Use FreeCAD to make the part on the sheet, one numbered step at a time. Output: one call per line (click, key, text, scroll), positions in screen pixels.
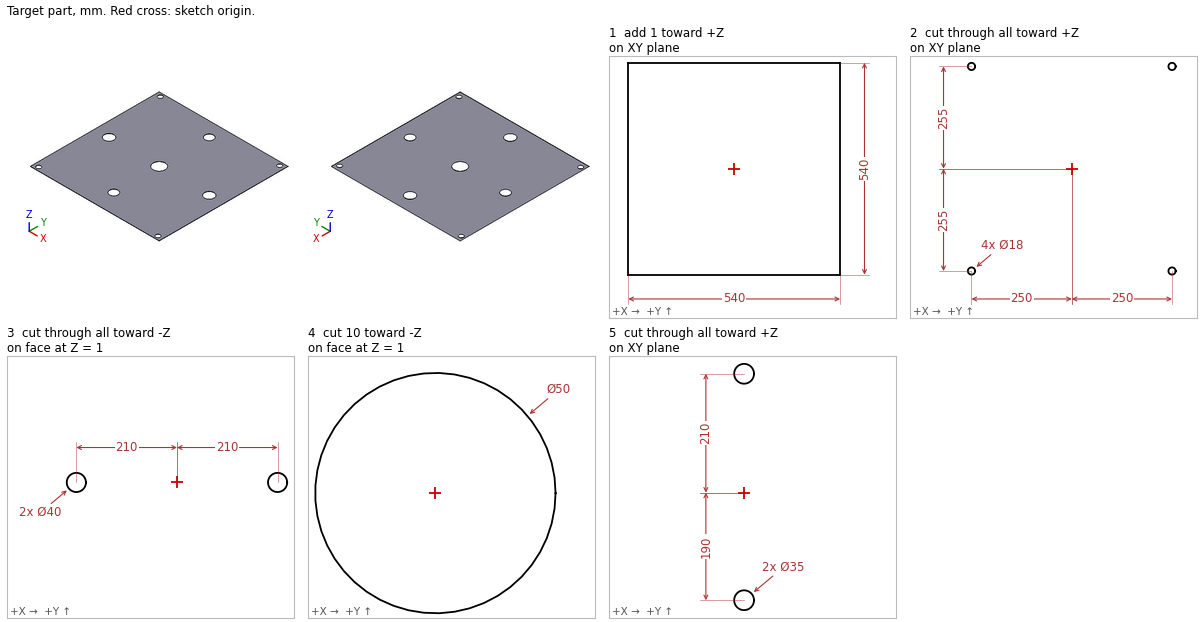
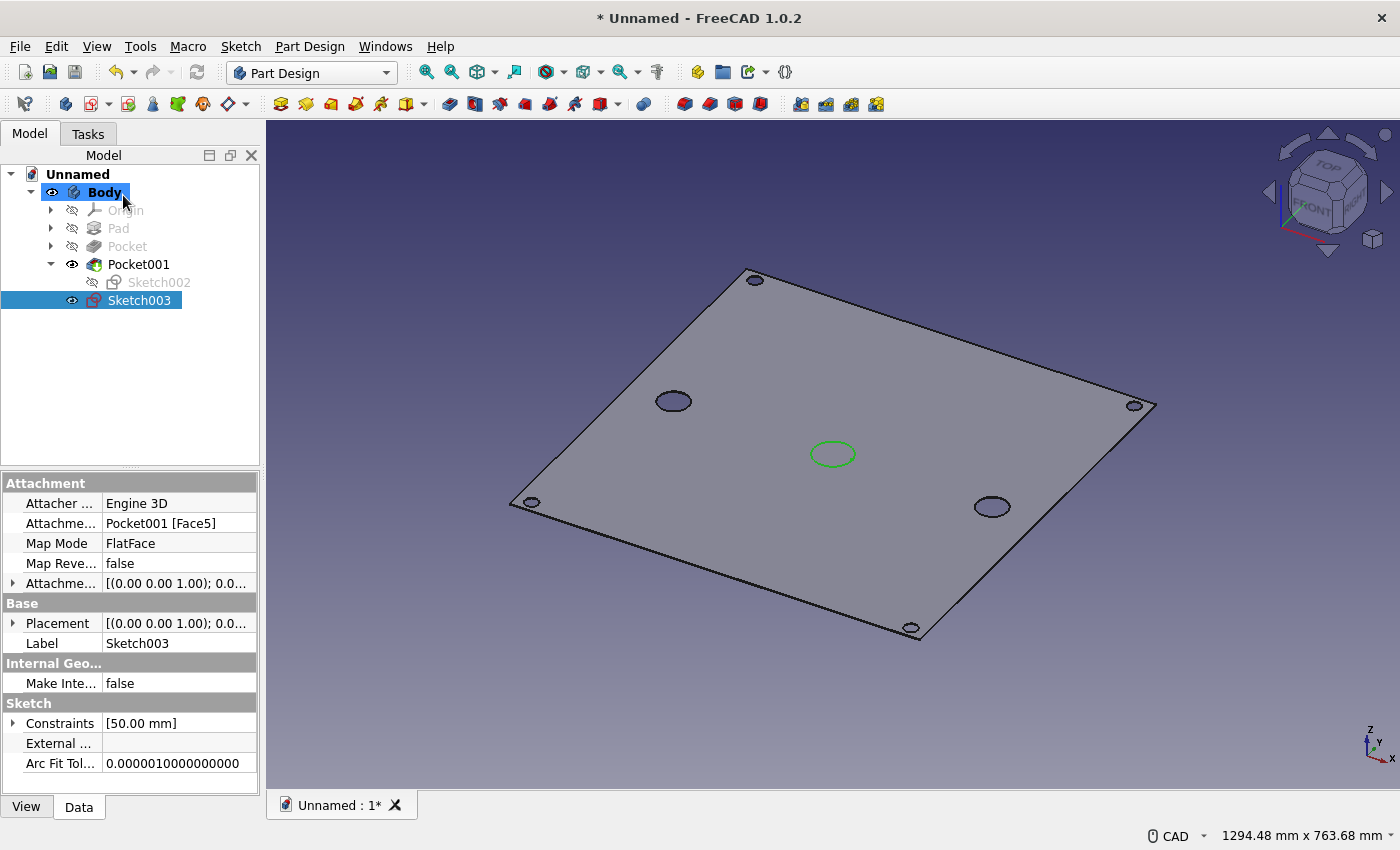
click(450, 104)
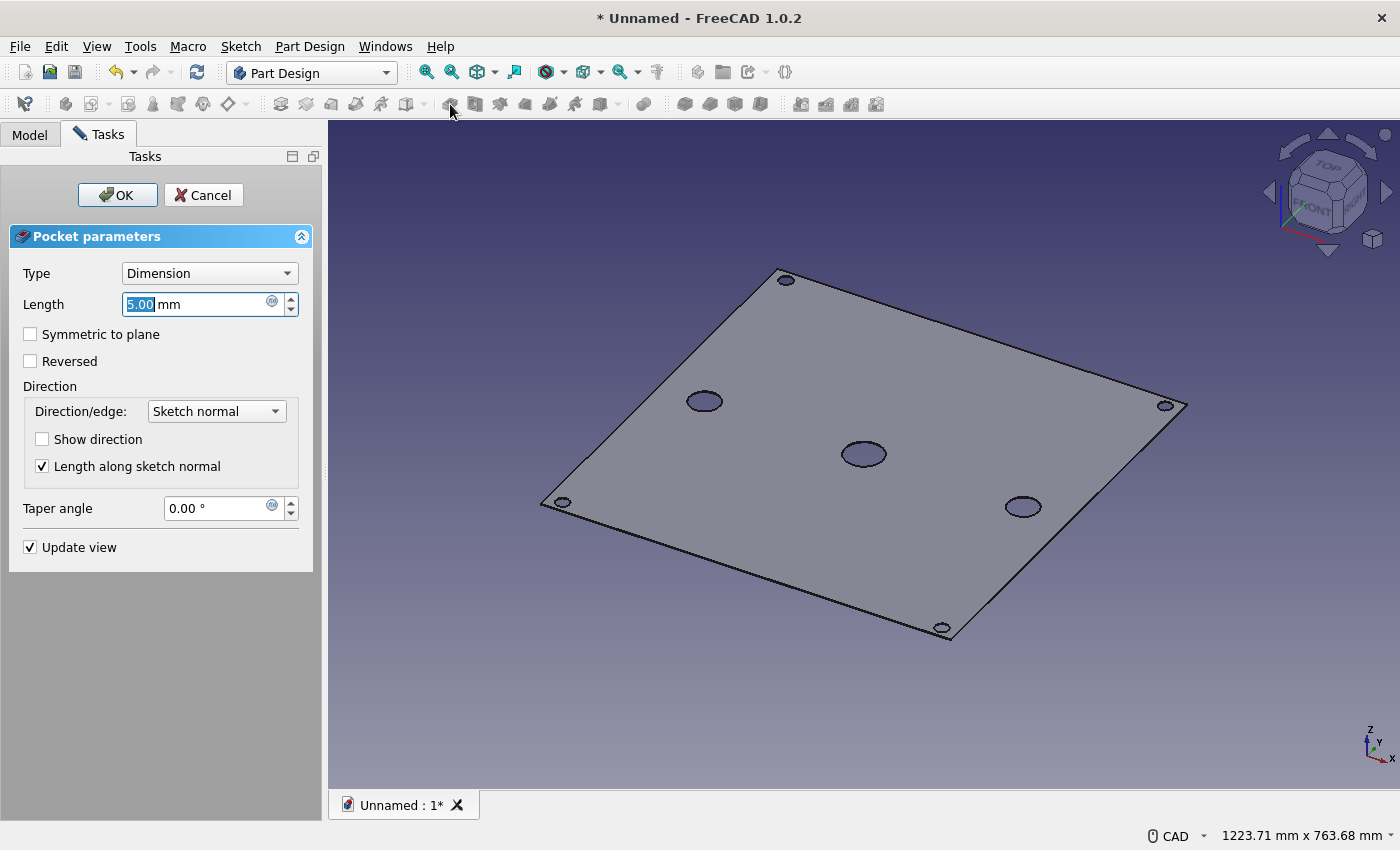
text(10)
key(Tab)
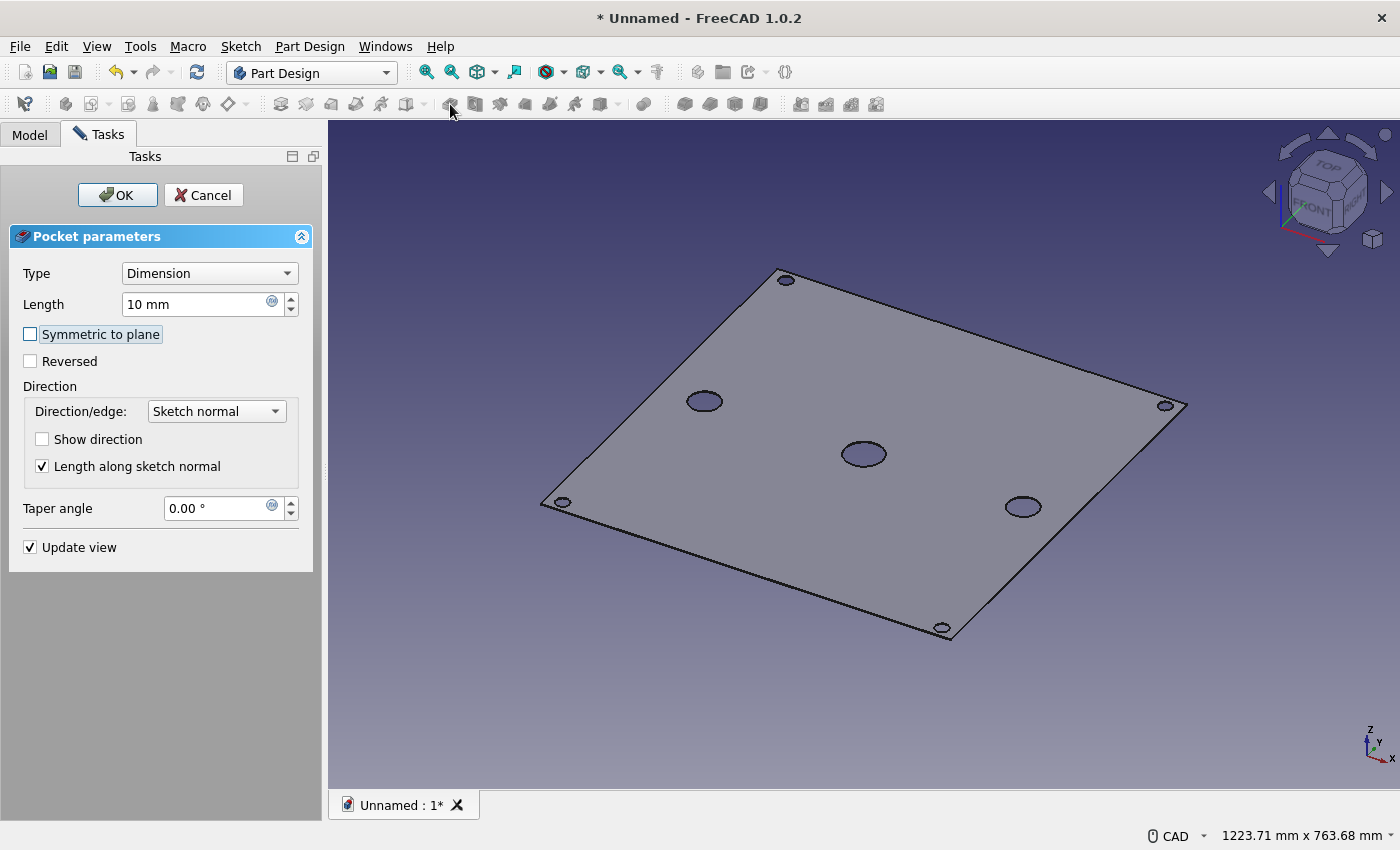
click(118, 195)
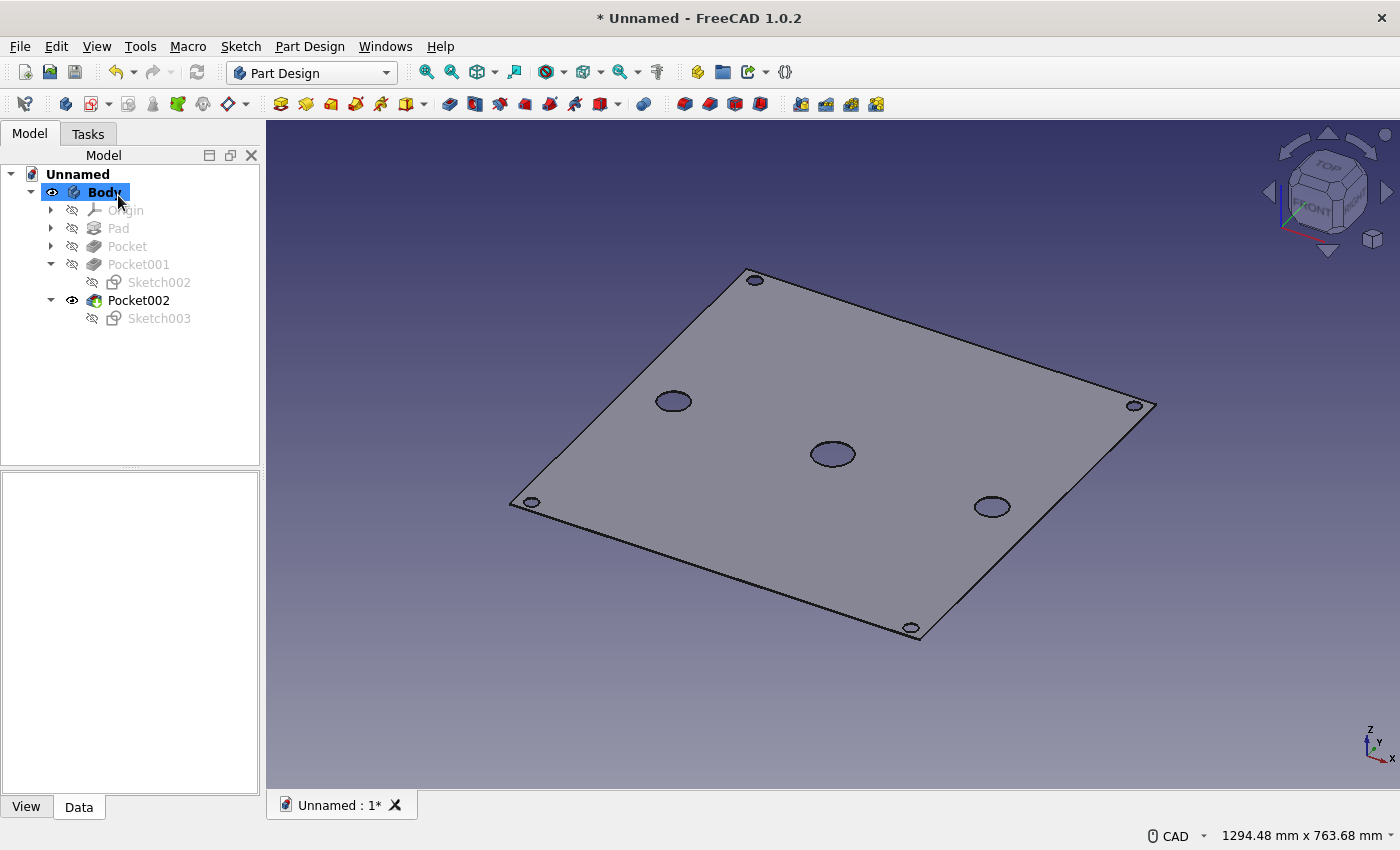
click(90, 104)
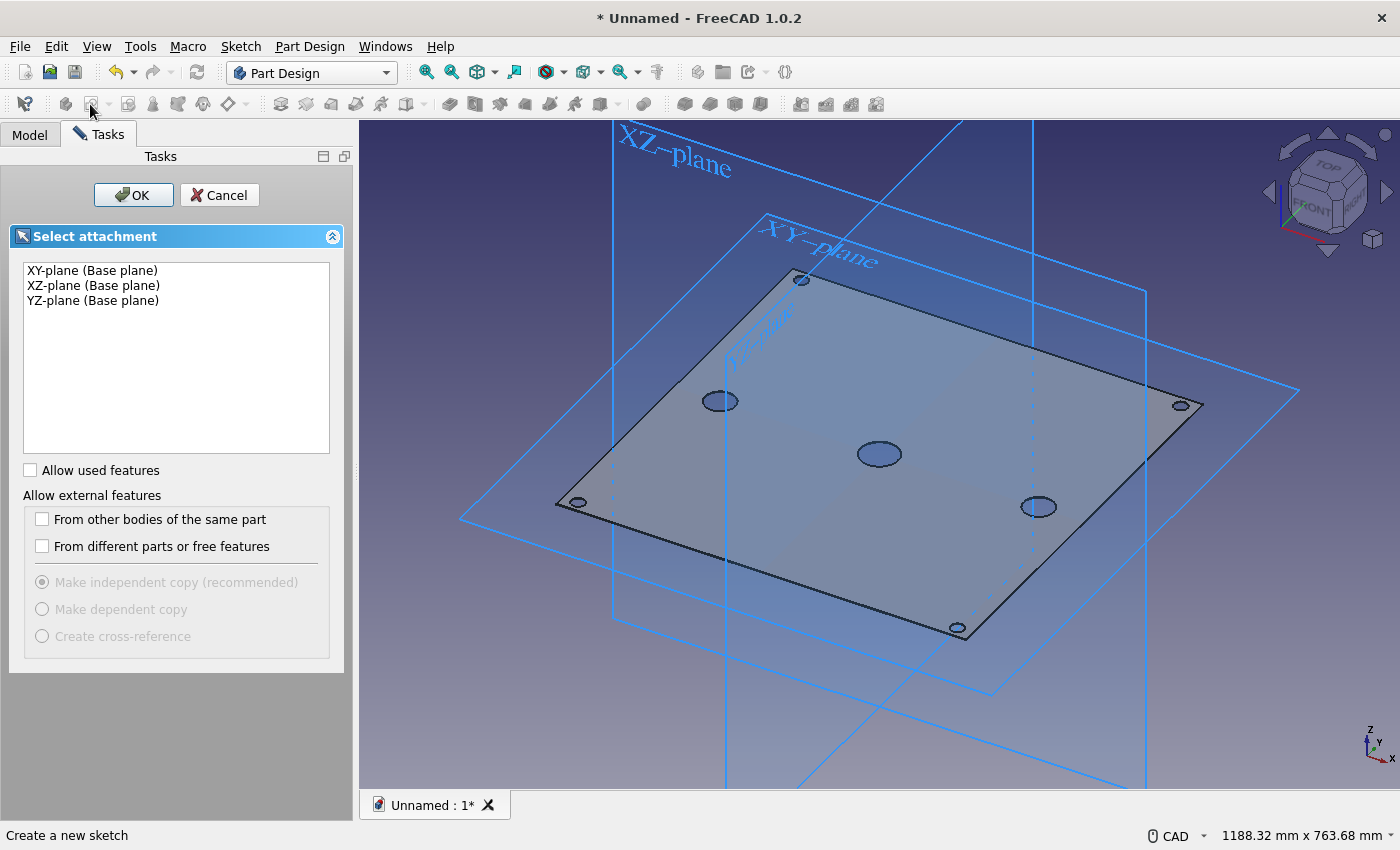
click(84, 270)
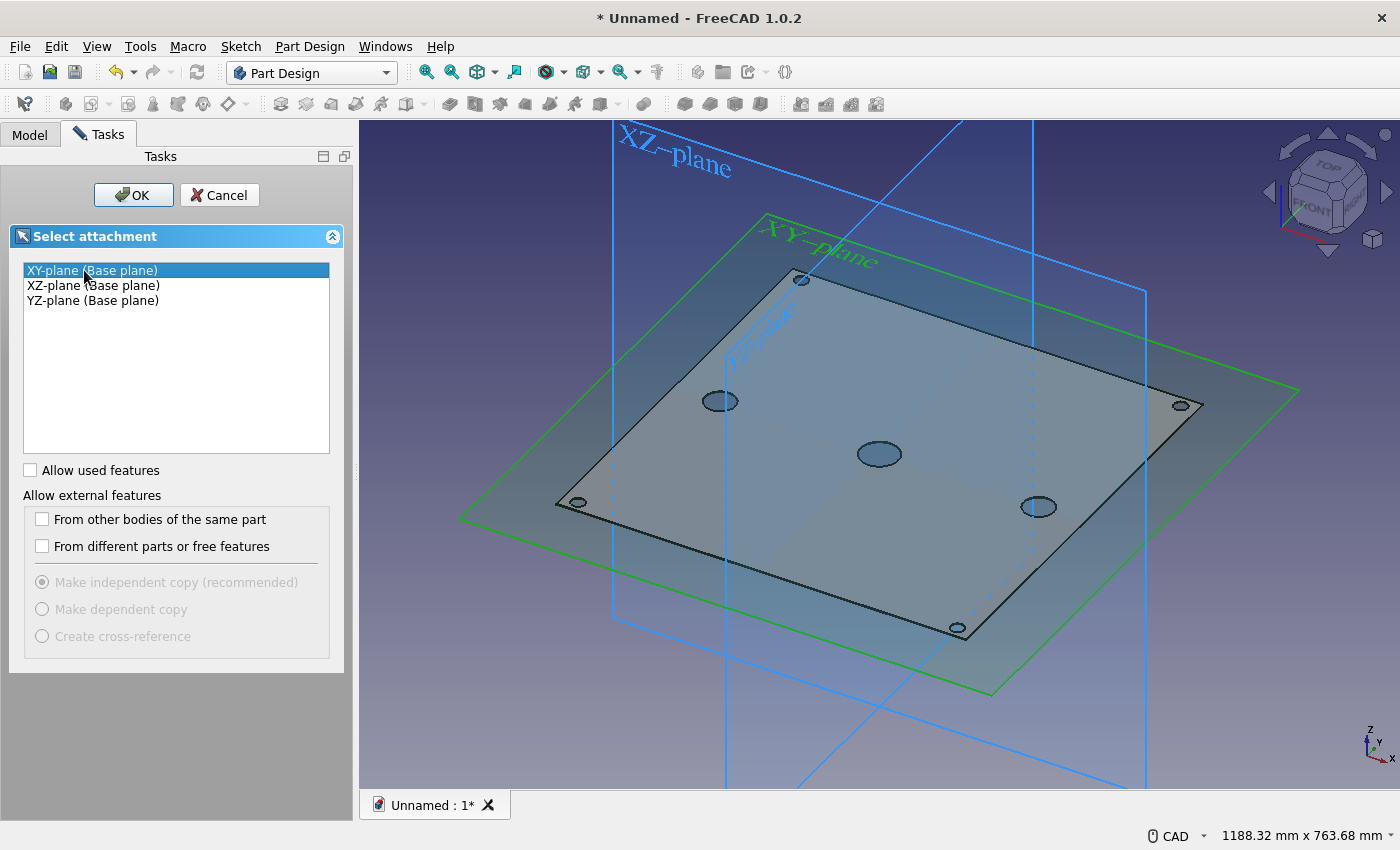
click(134, 195)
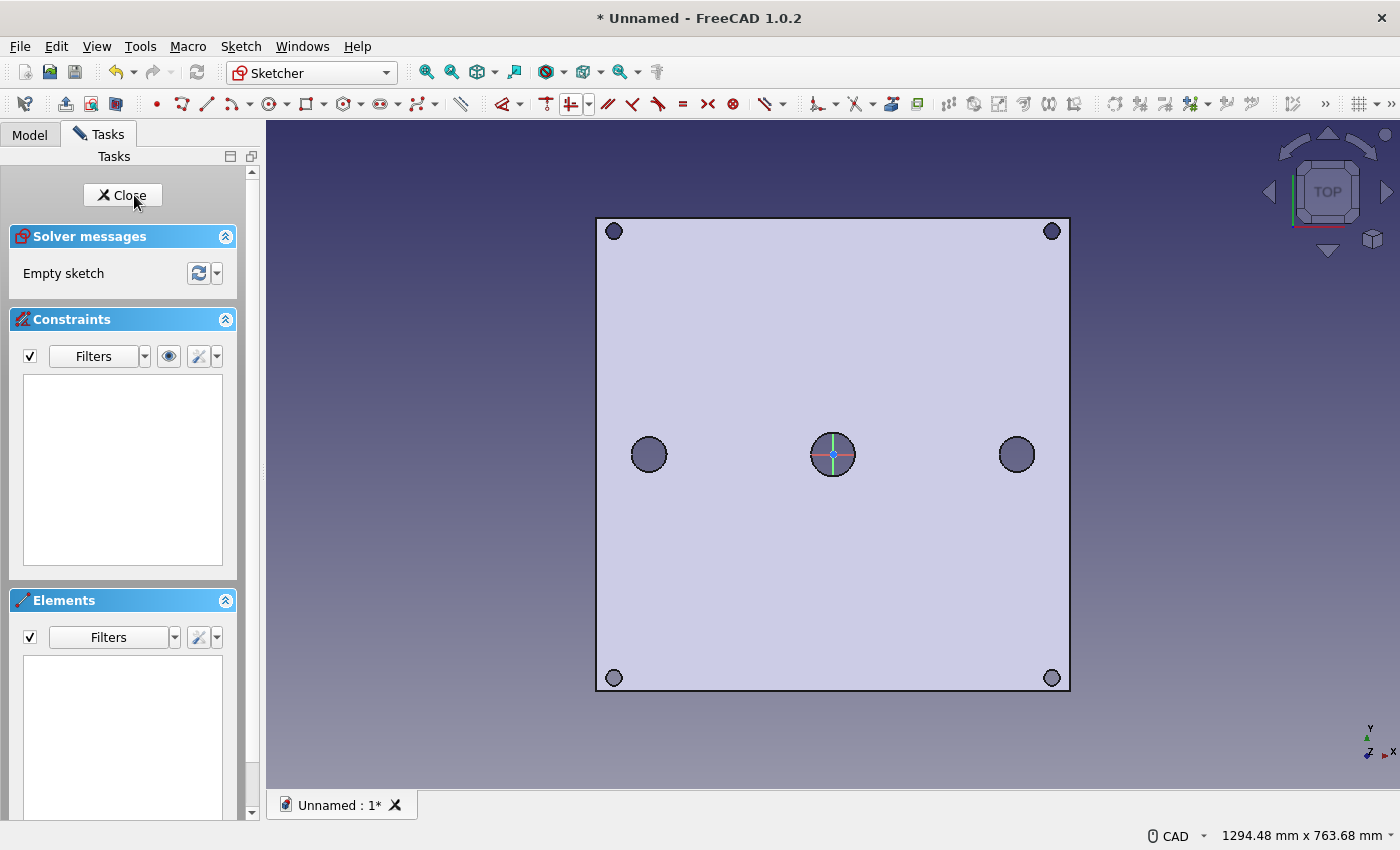
key(q)
key(s)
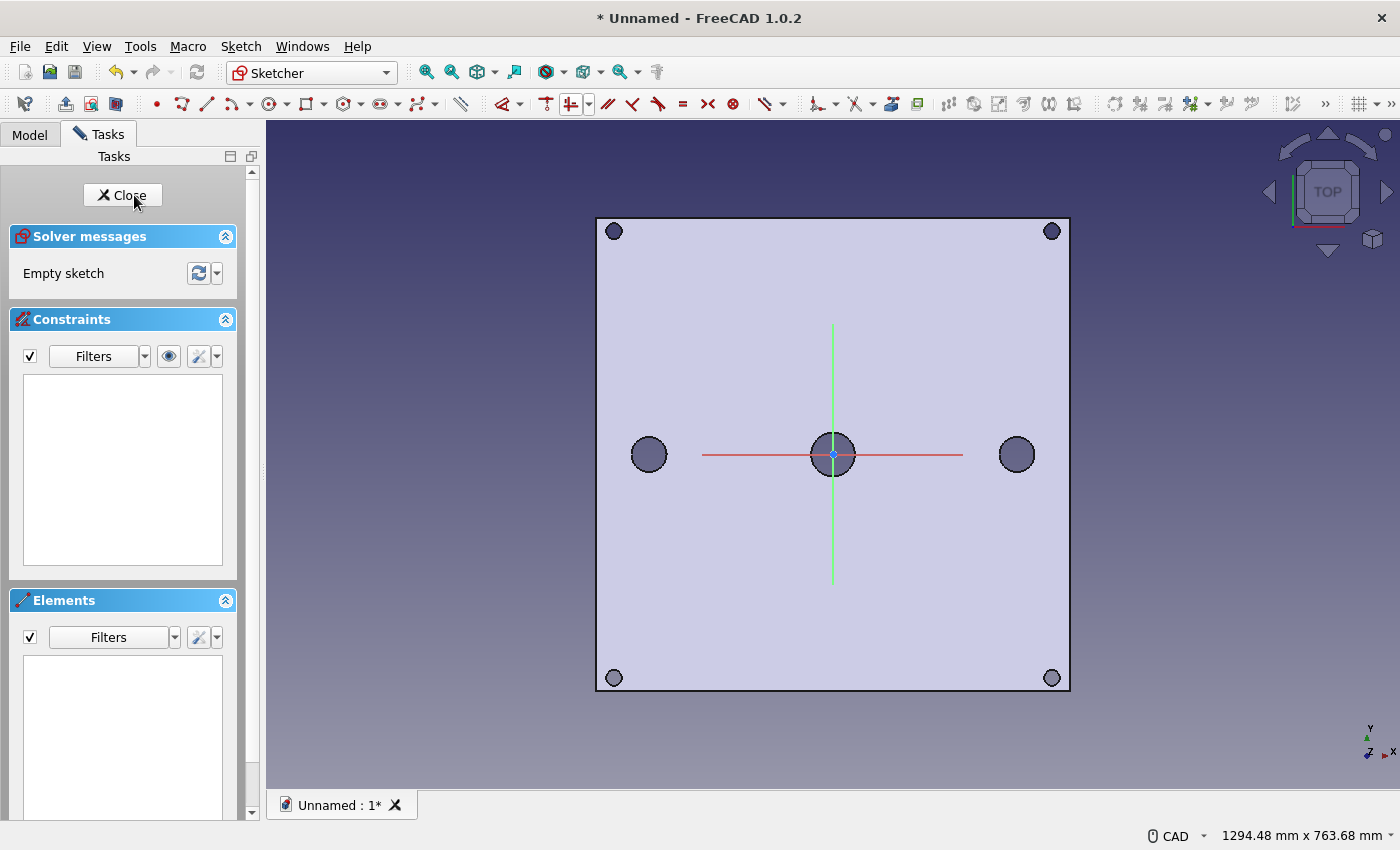
click(268, 104)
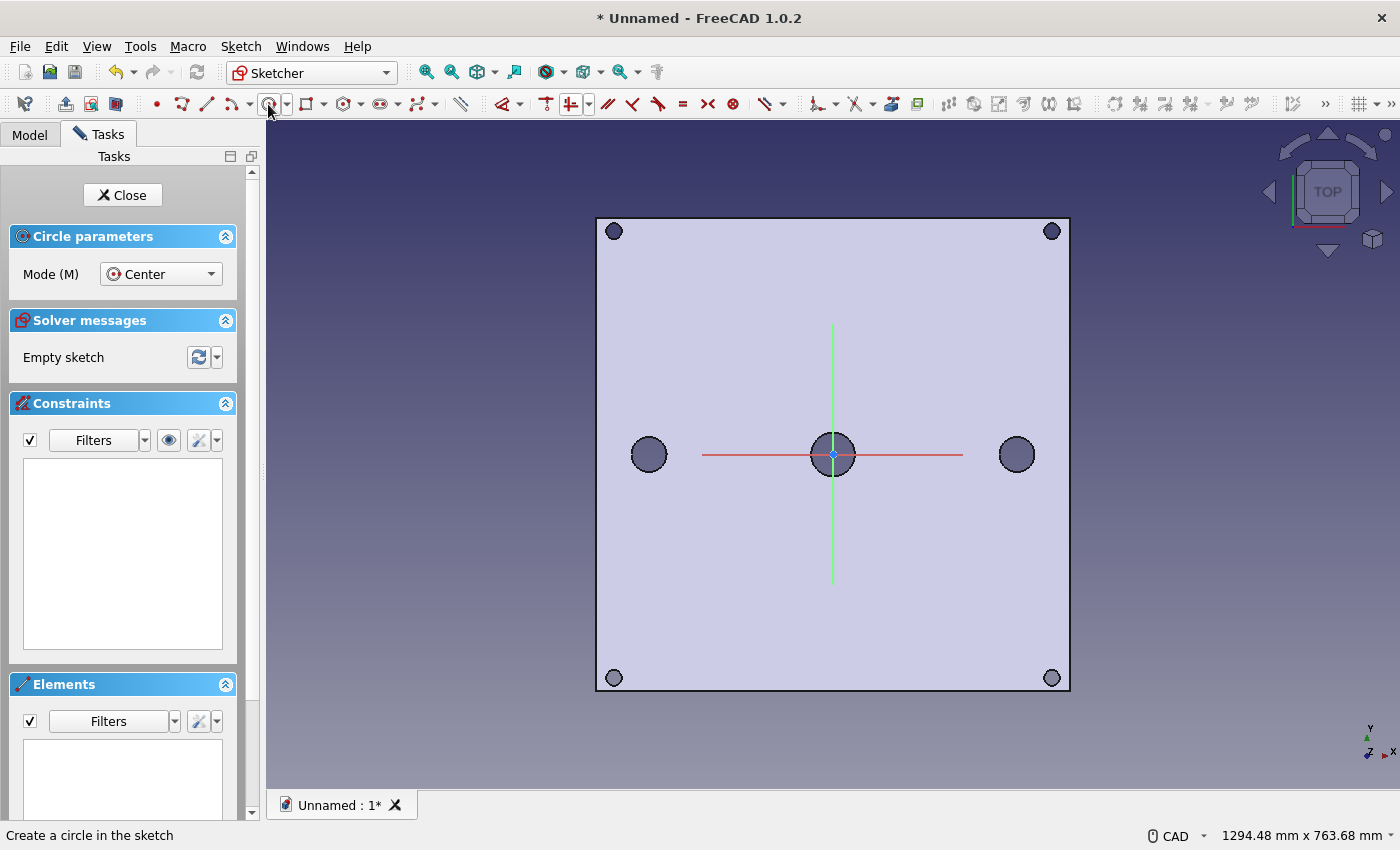
scroll(833, 621, up, 2)